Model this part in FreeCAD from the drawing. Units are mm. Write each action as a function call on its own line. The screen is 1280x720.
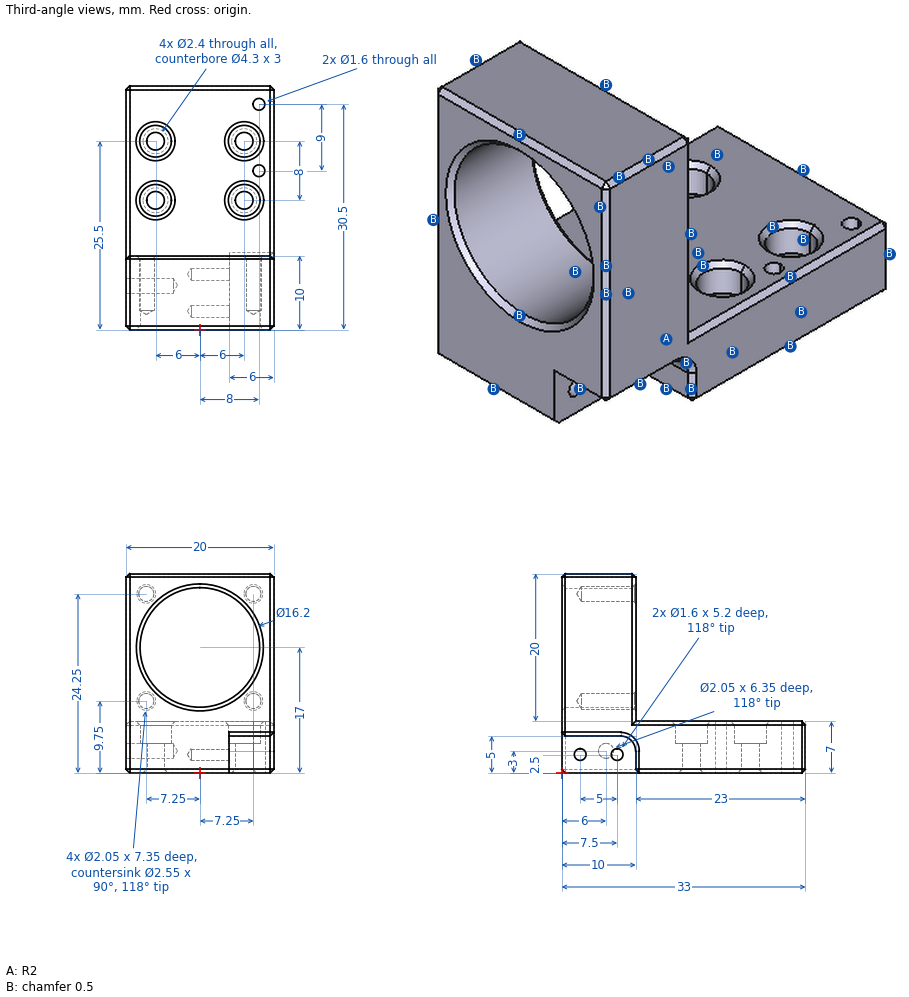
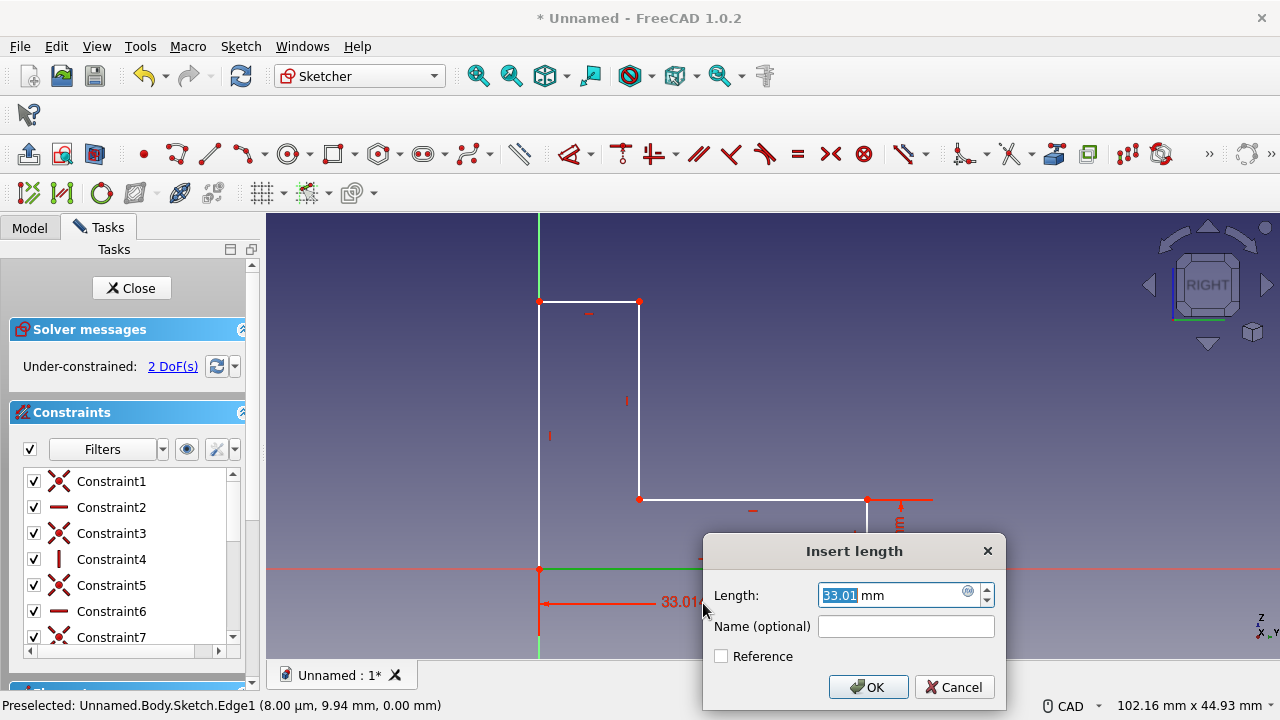
text(33)
key(Return)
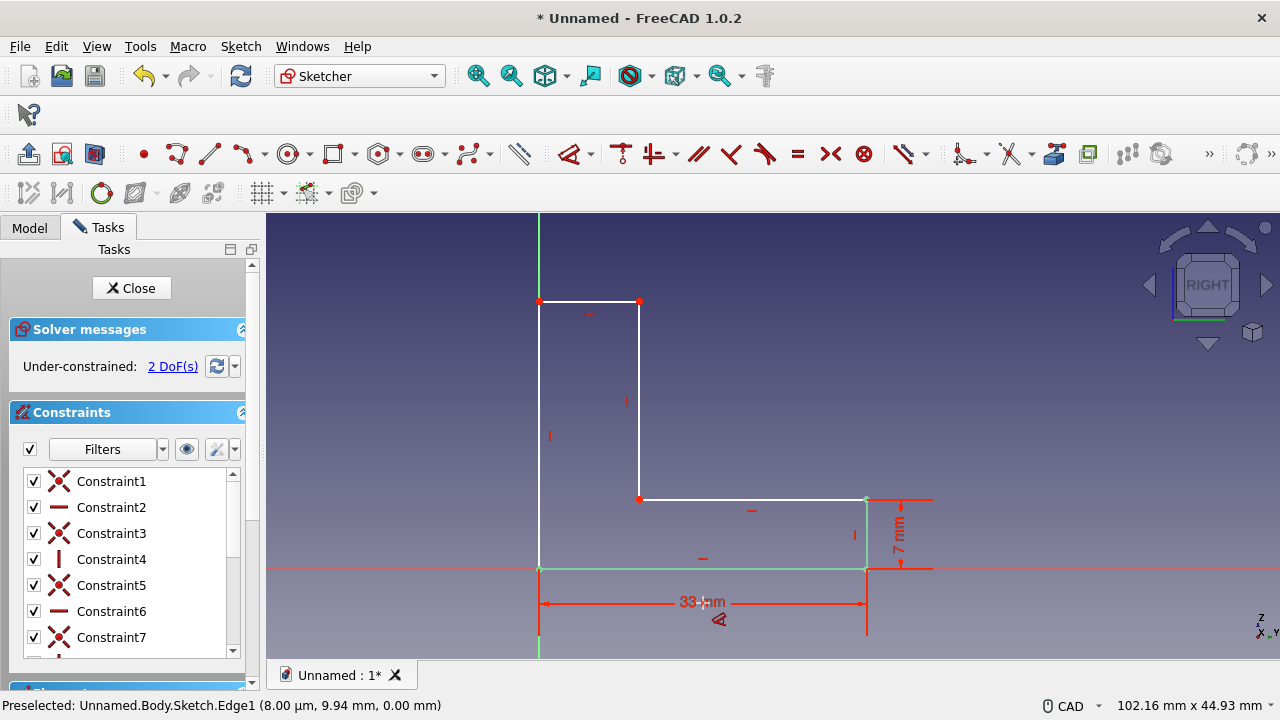
click(799, 500)
click(753, 534)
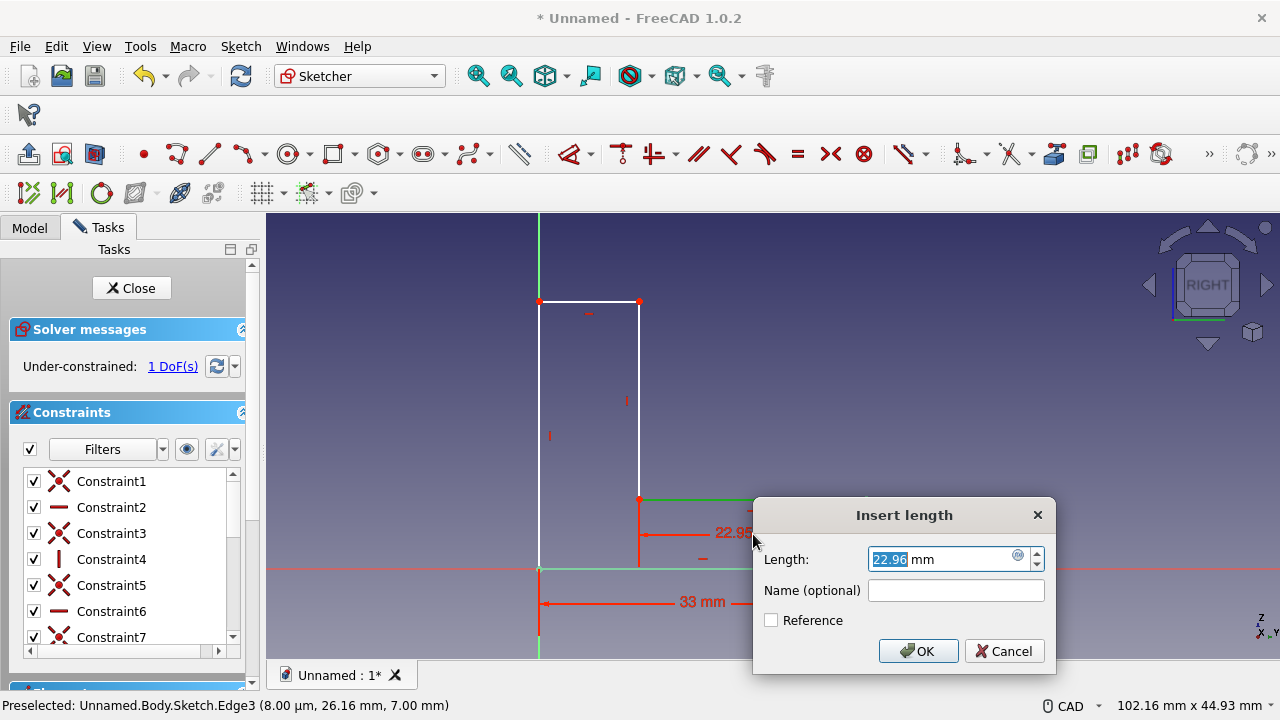
text(23)
key(Return)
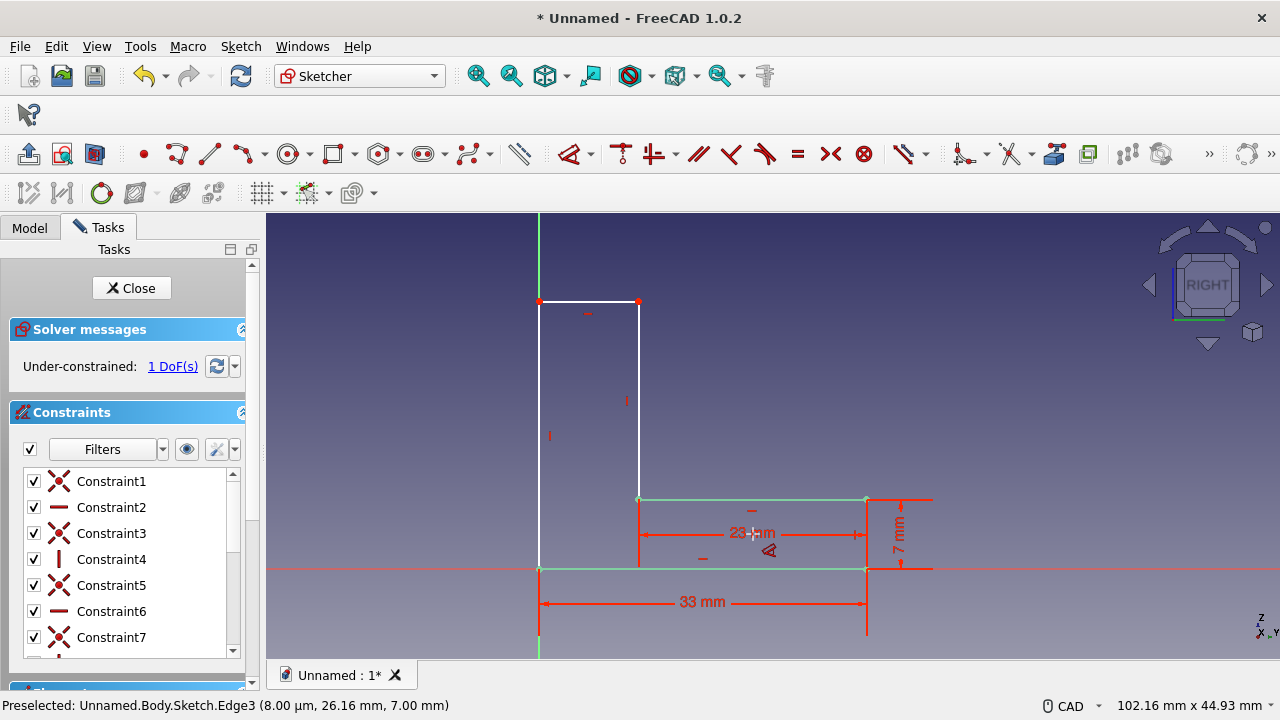
click(639, 440)
click(605, 401)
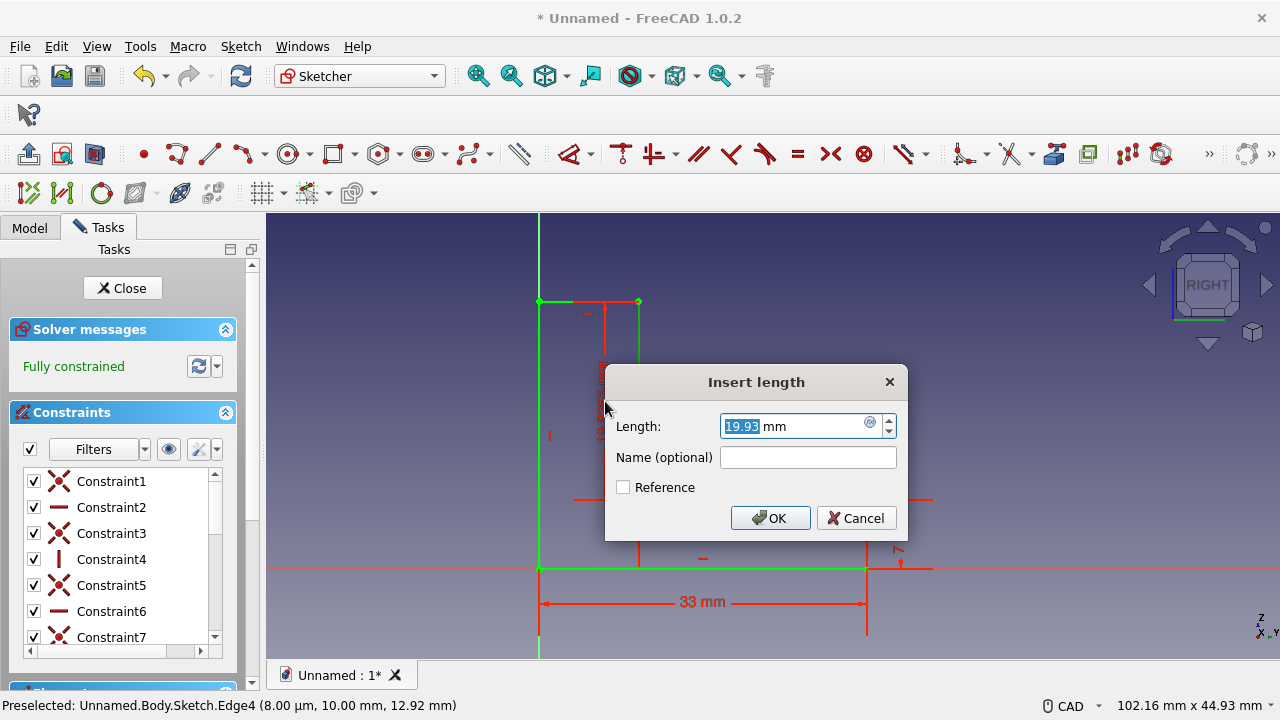
text(20)
key(Return)
key(Escape)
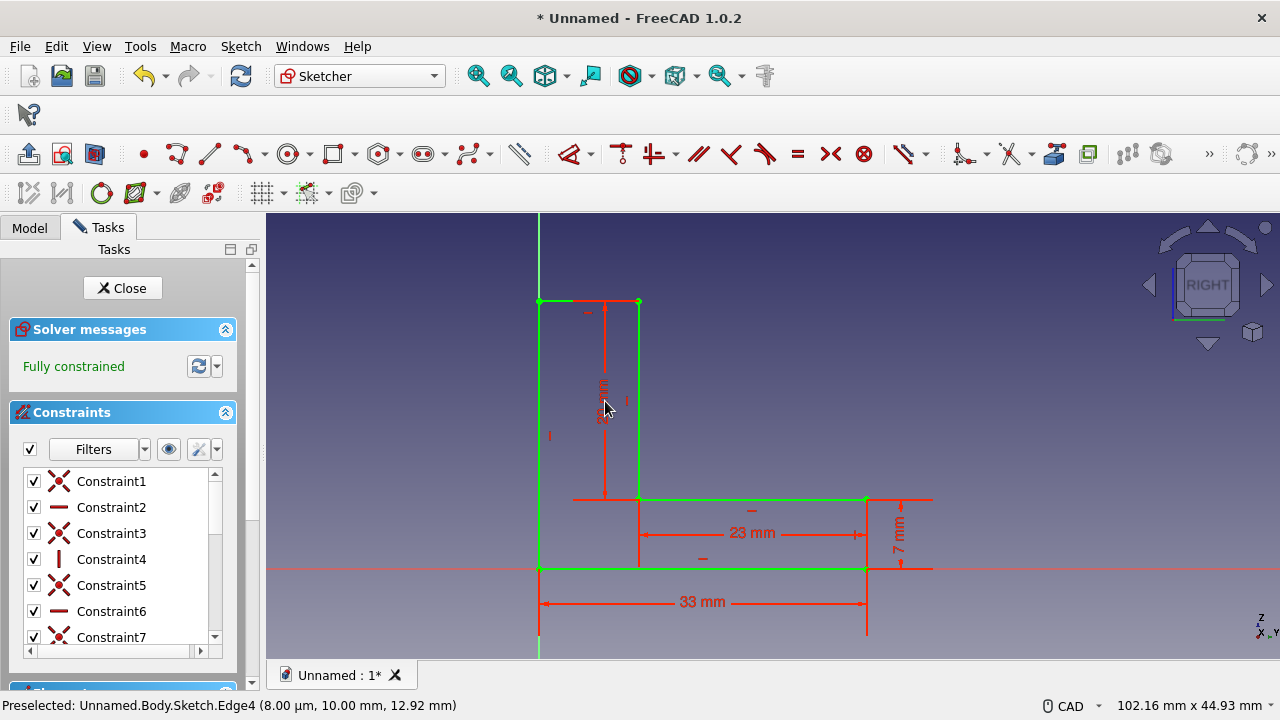
click(123, 288)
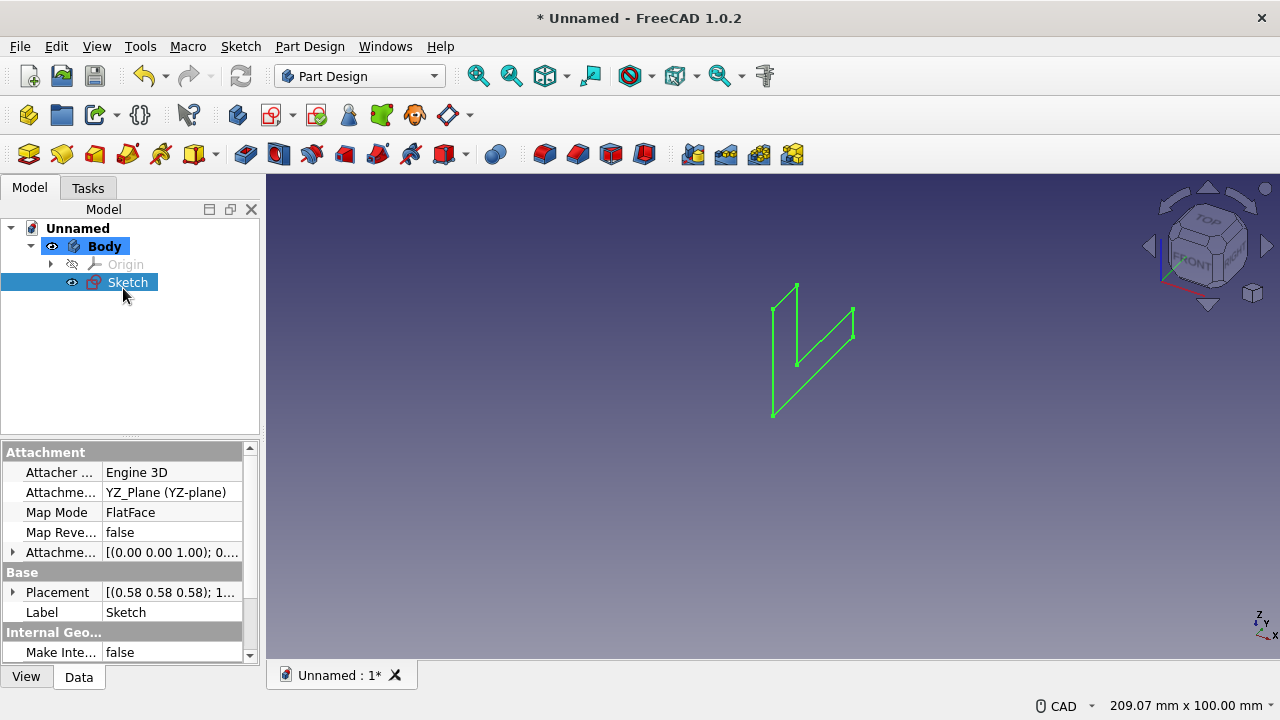
click(29, 154)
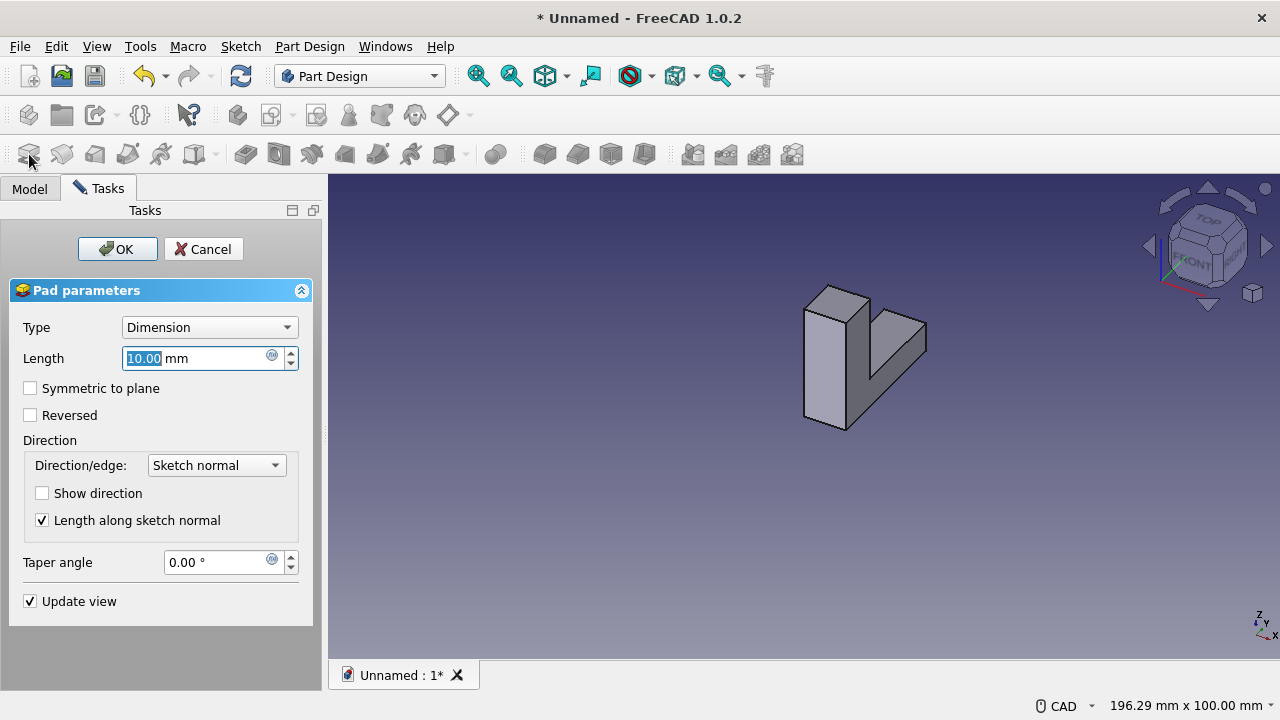
text(20)
key(Tab)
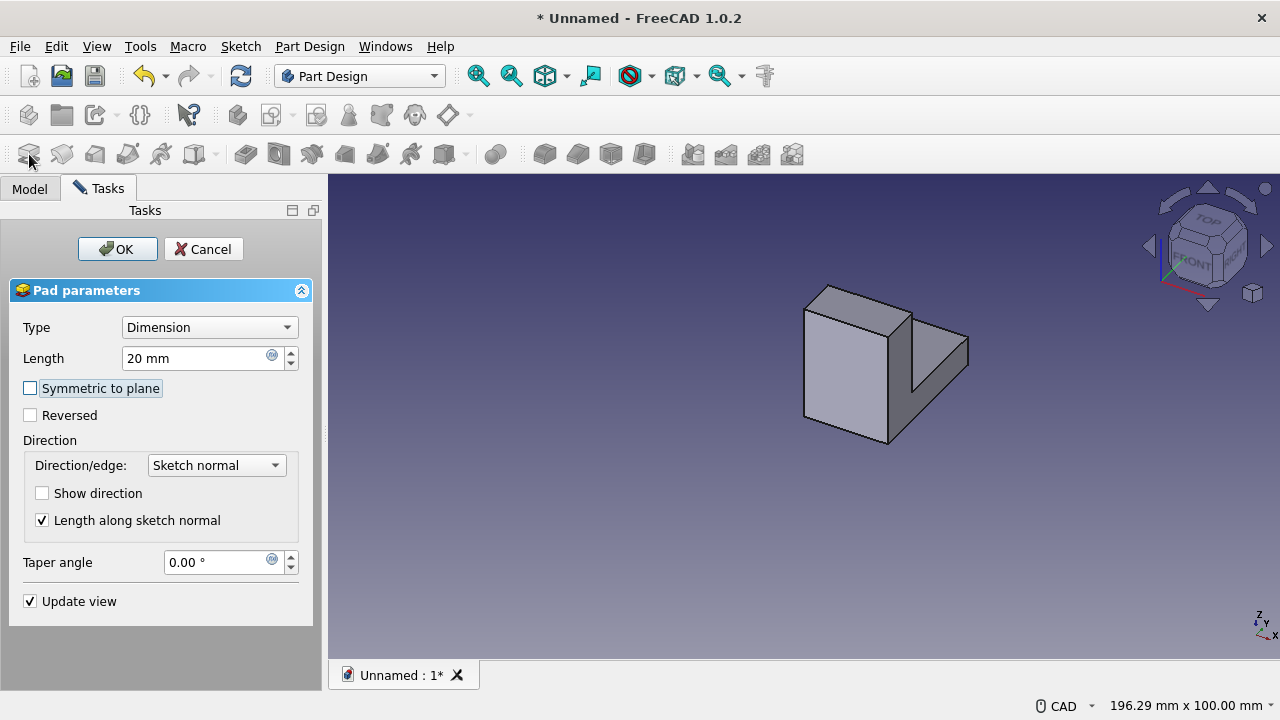
click(31, 388)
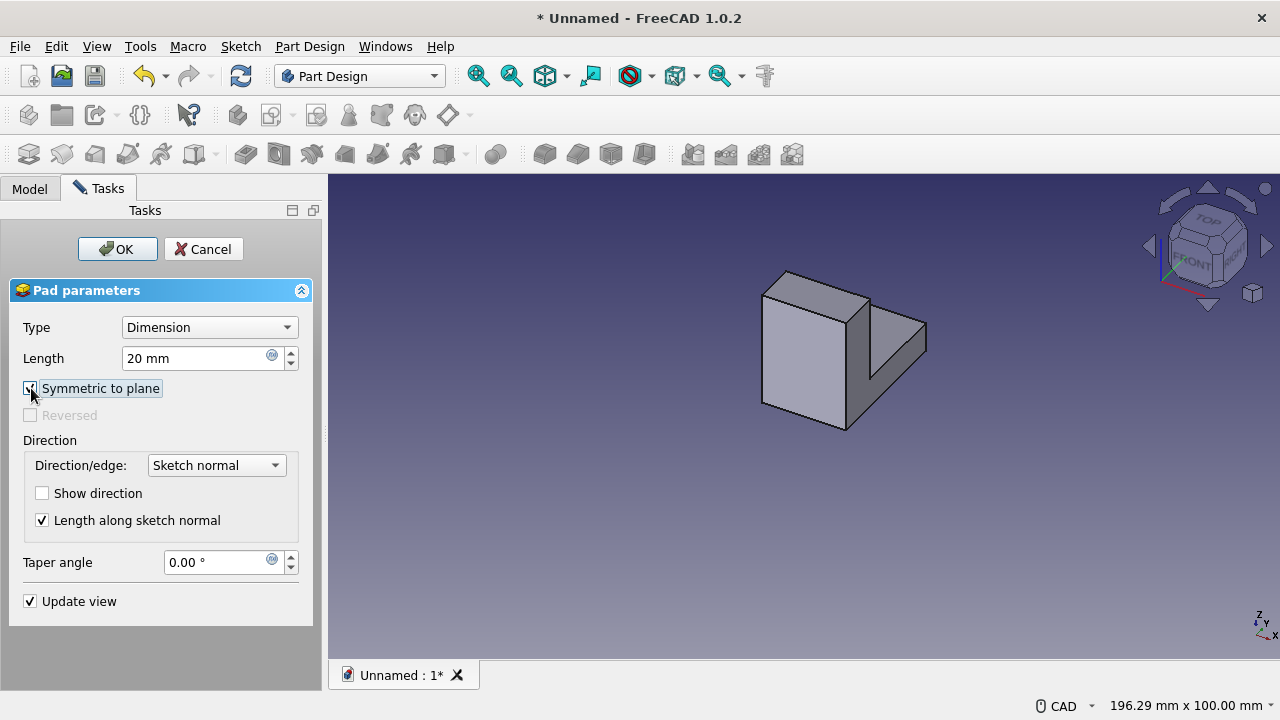
click(118, 249)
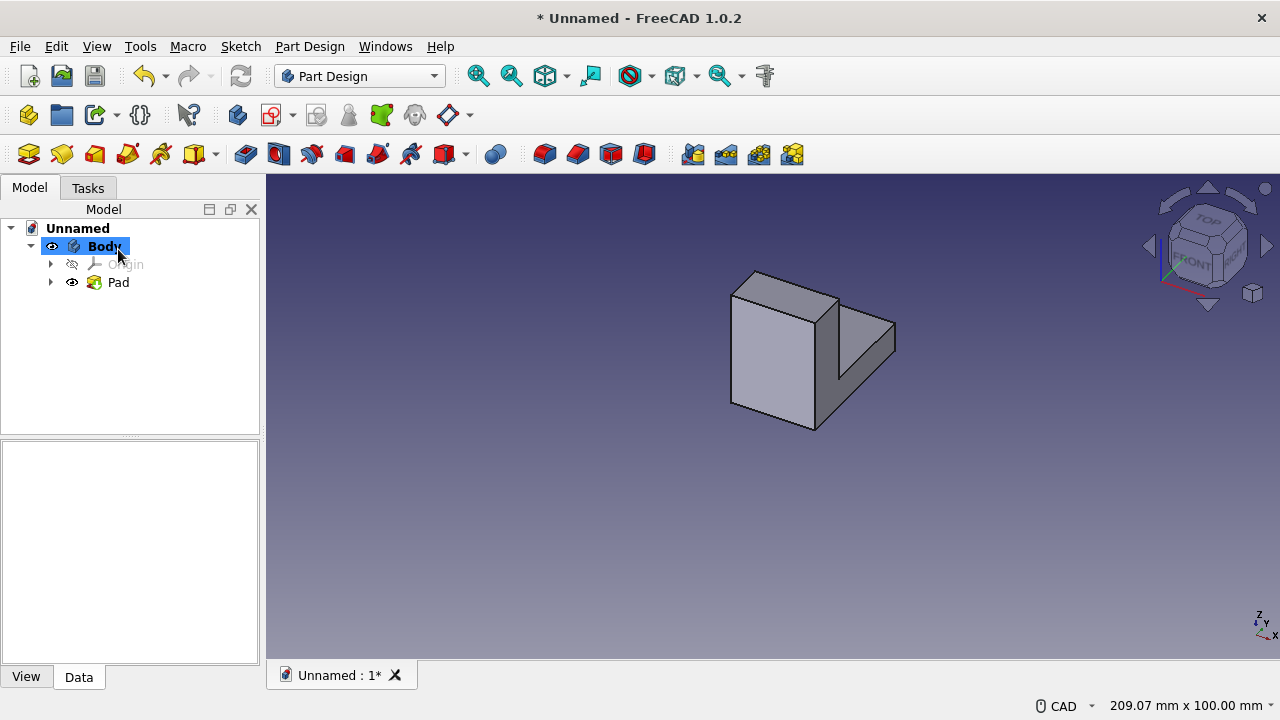
click(479, 76)